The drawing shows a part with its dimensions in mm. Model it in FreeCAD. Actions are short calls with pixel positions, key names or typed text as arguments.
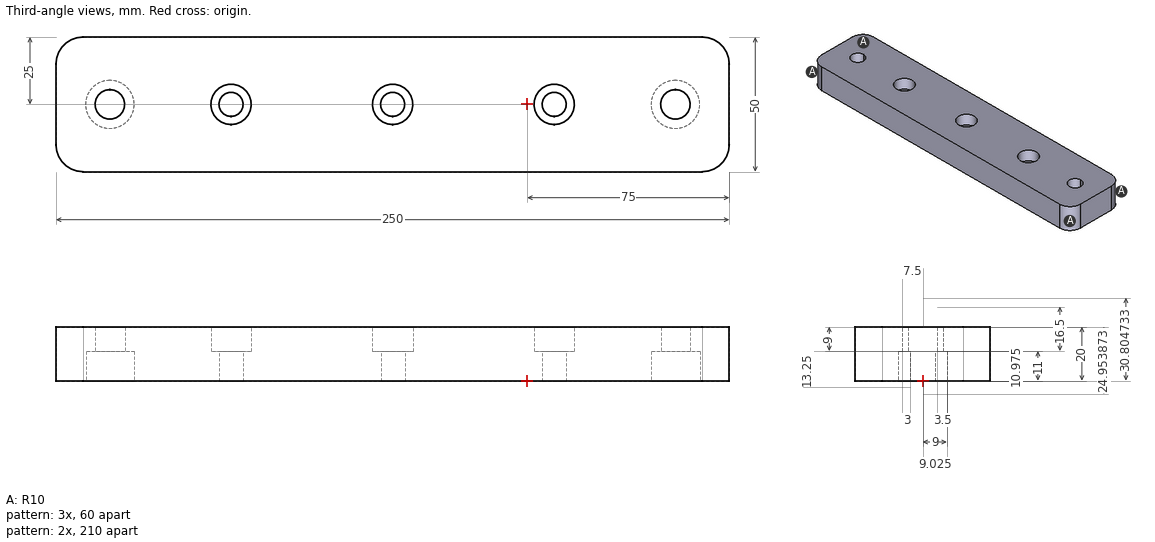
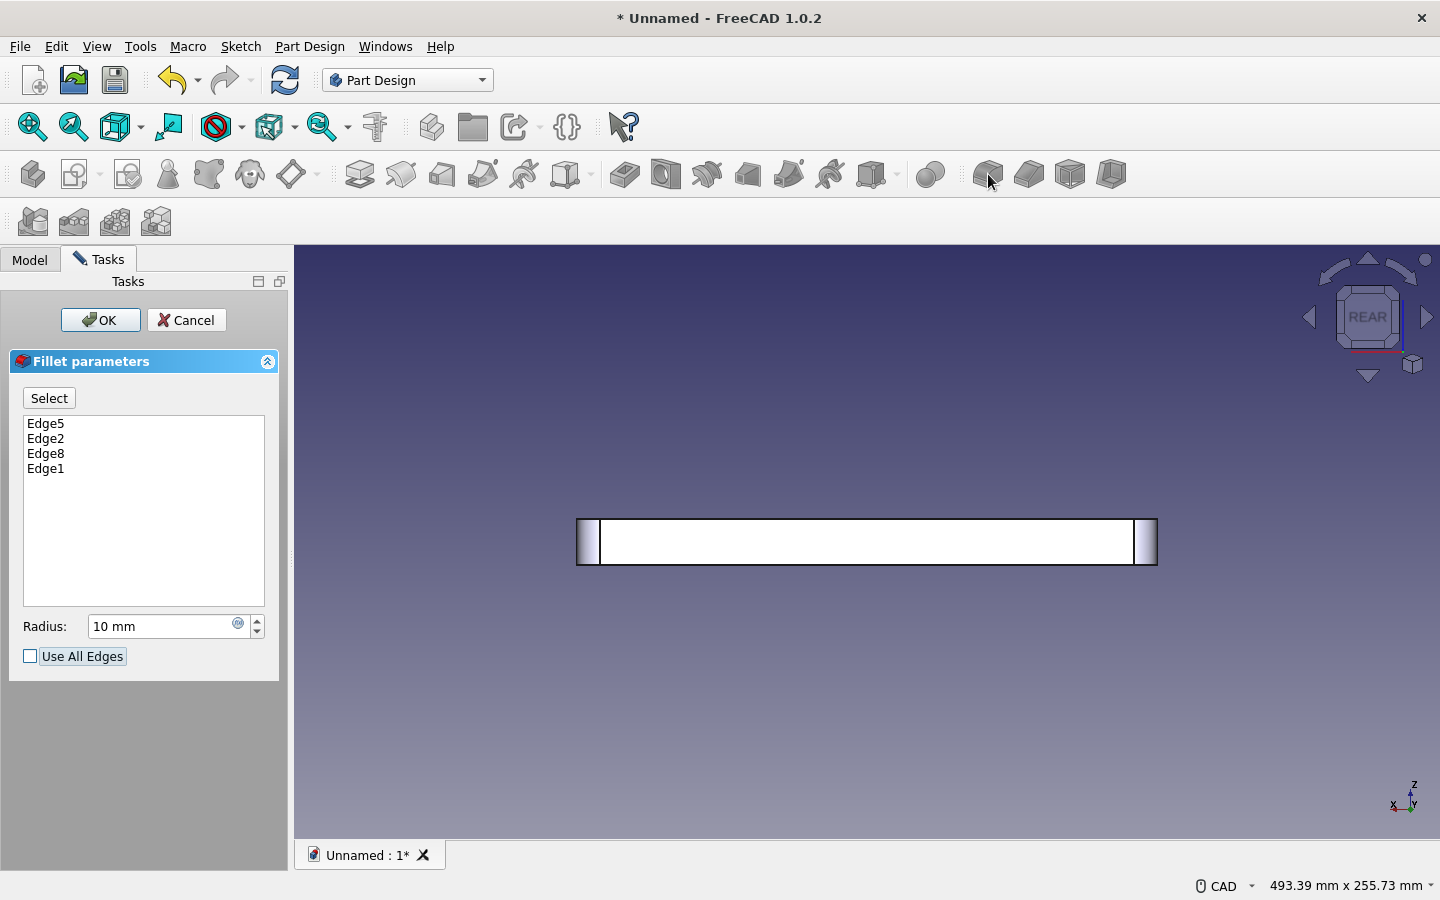
click(101, 320)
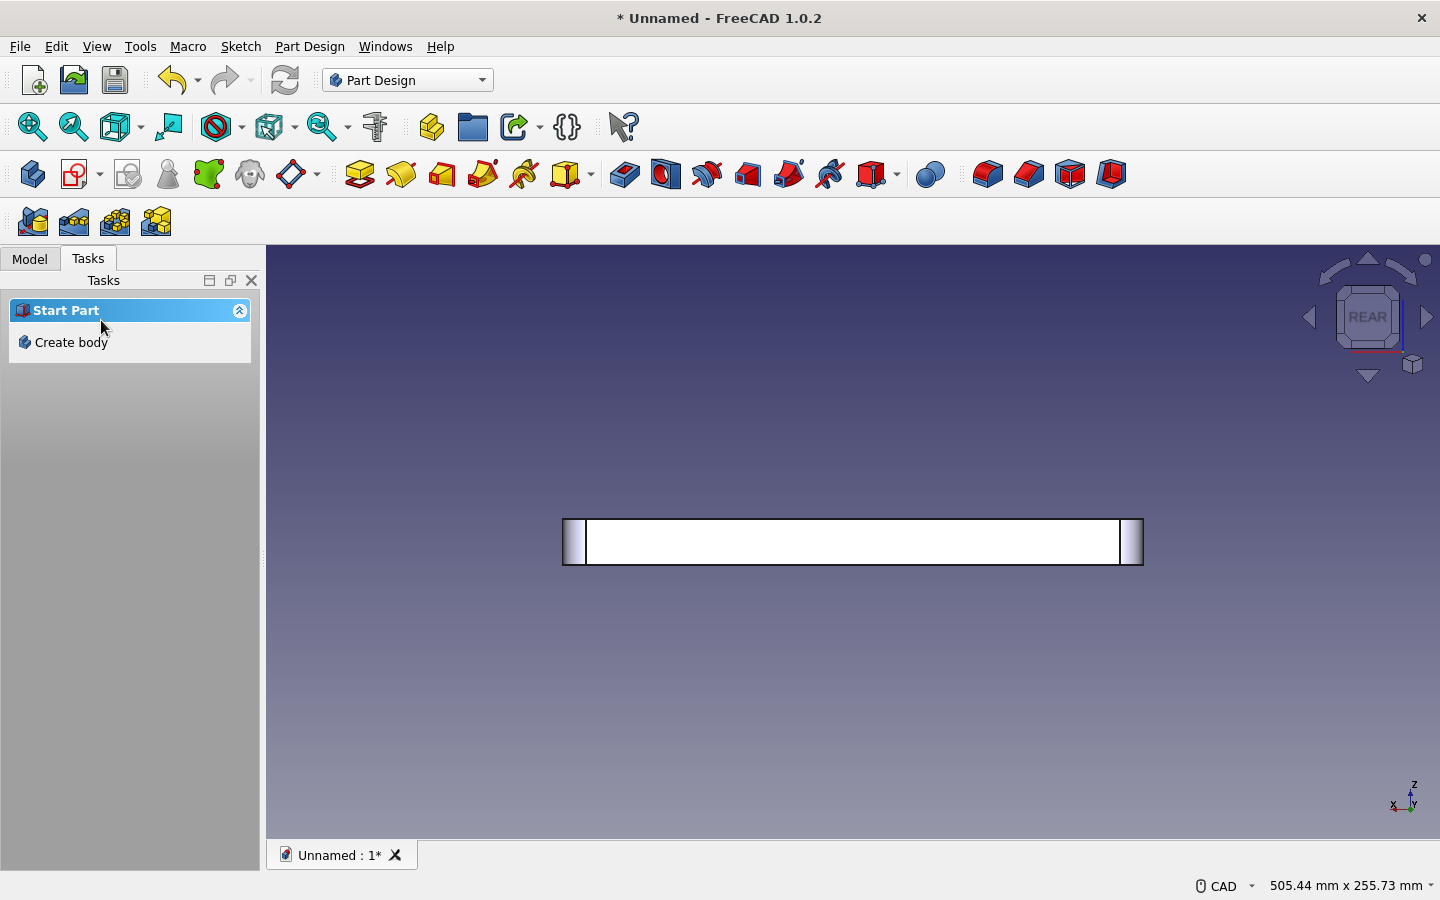
click(30, 258)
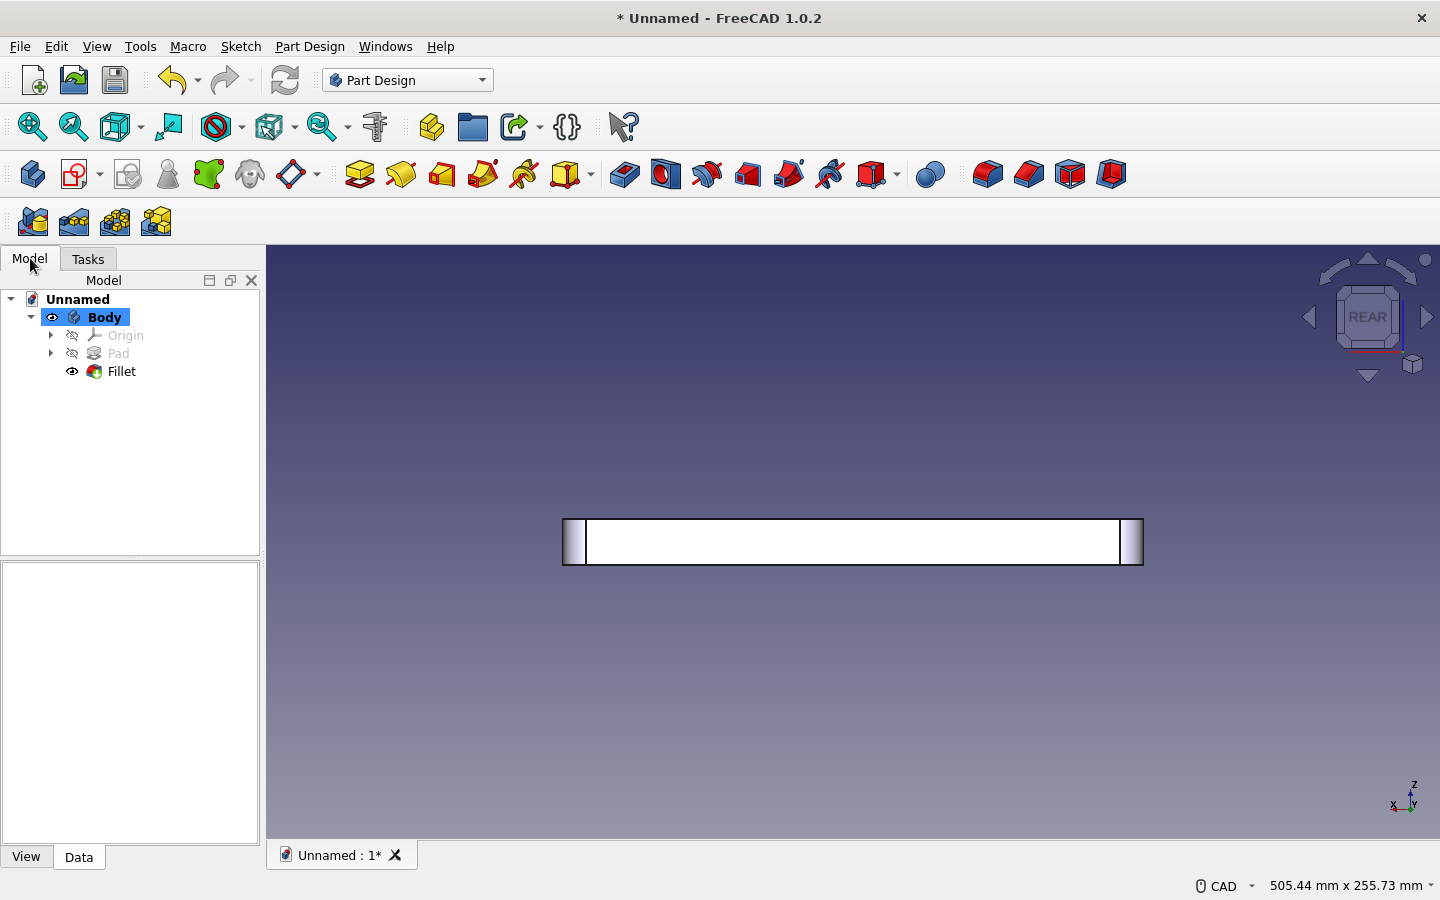
click(51, 335)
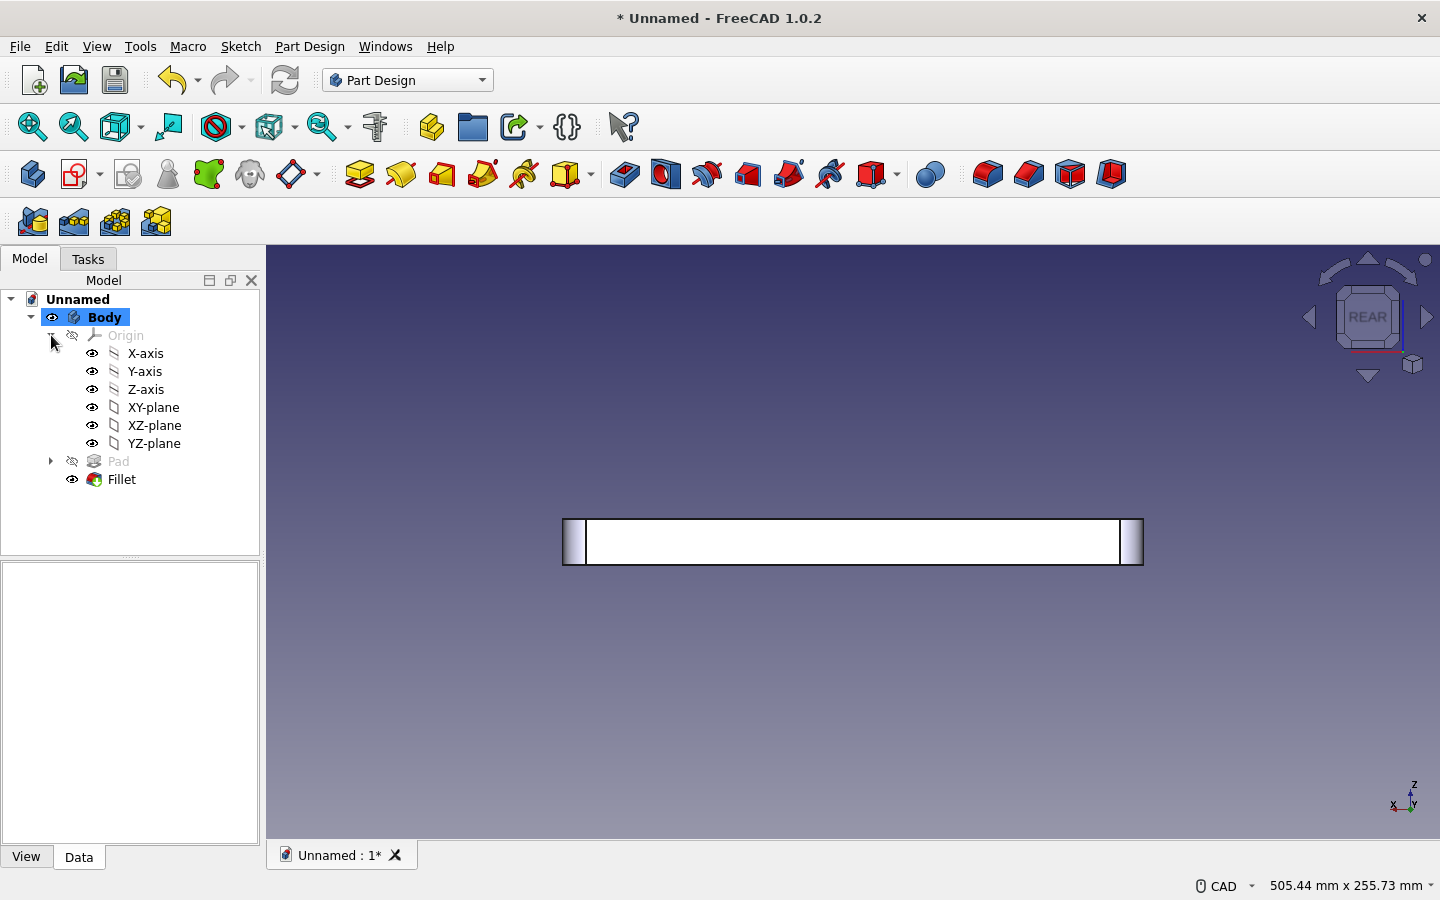
click(137, 443)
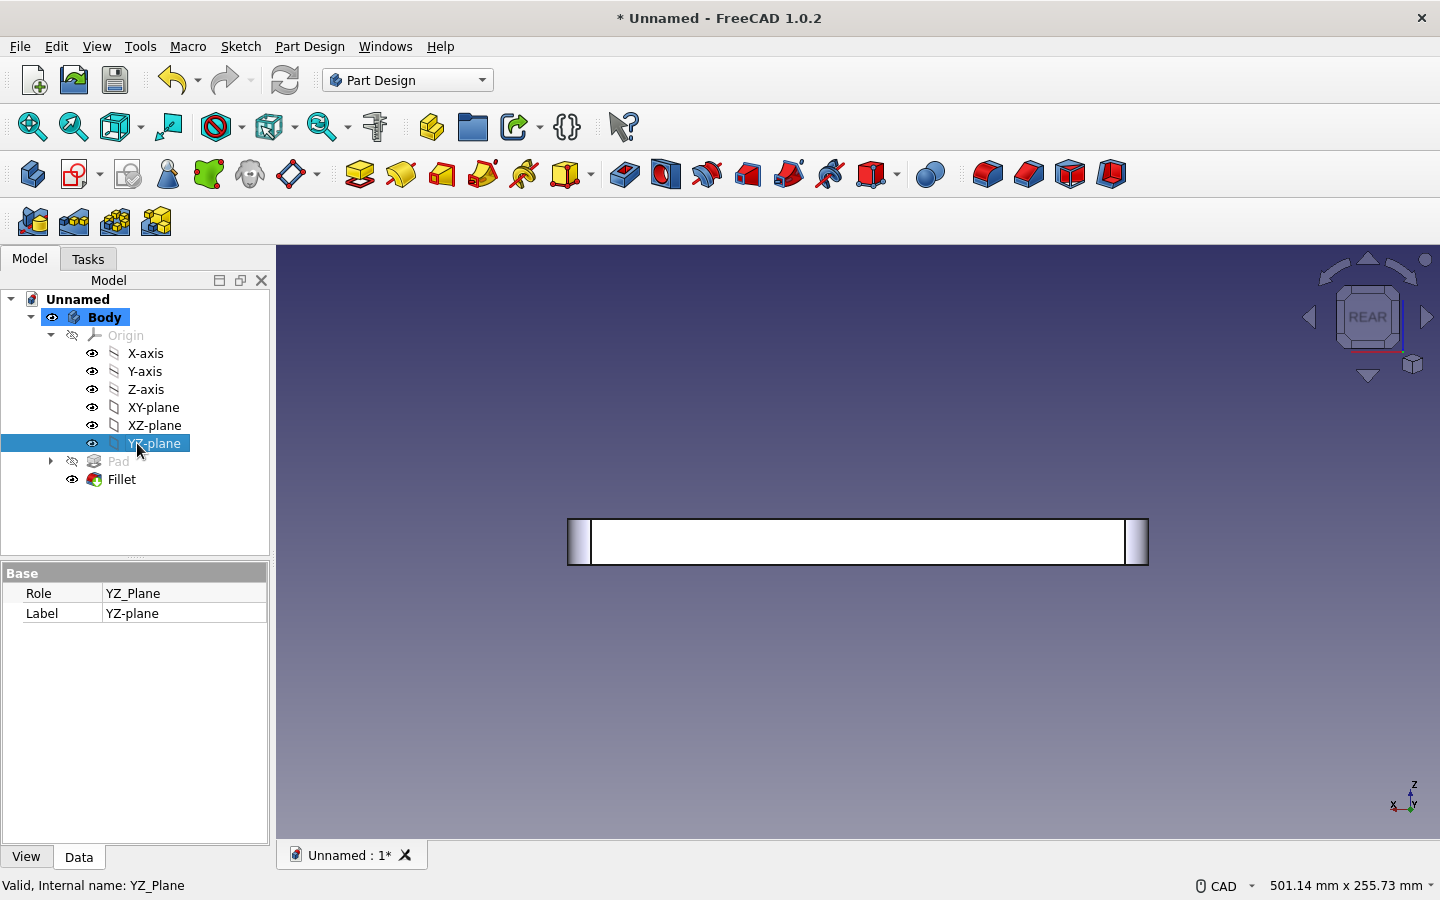
click(290, 174)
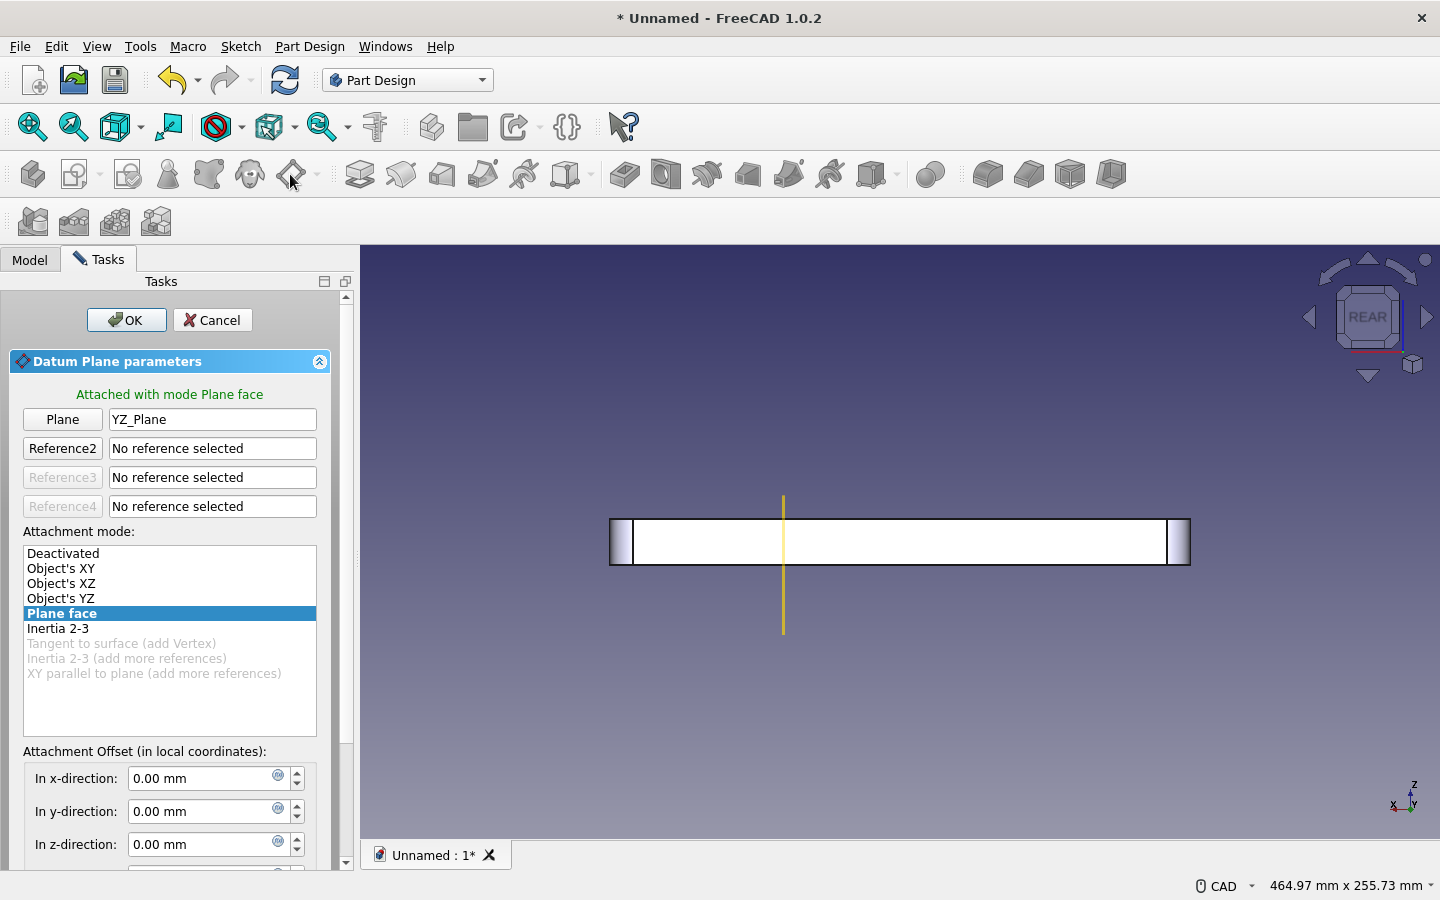
triple_click(210, 844)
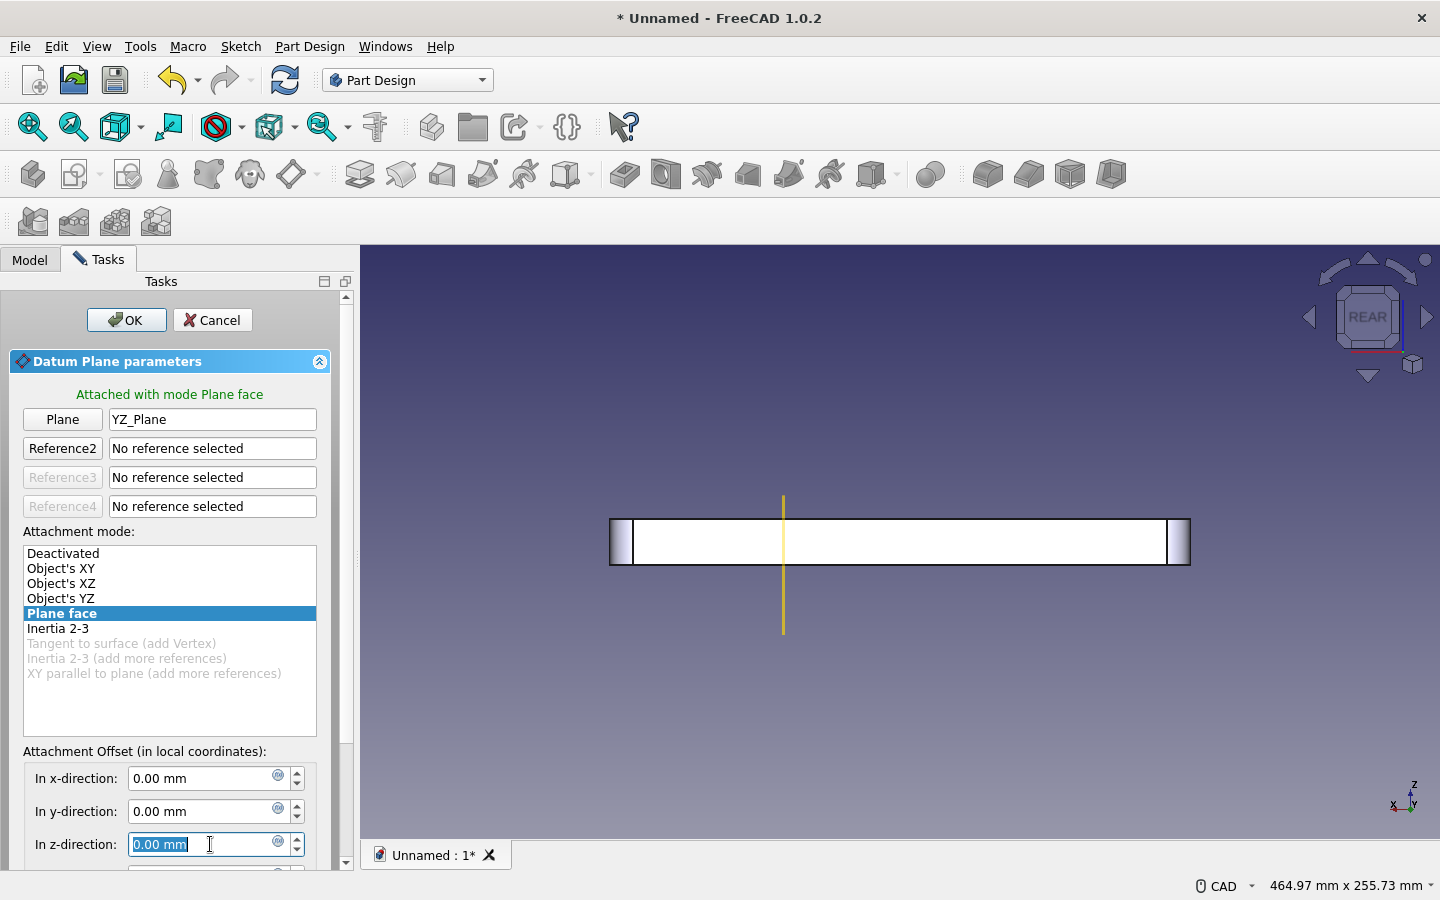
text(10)
key(Tab)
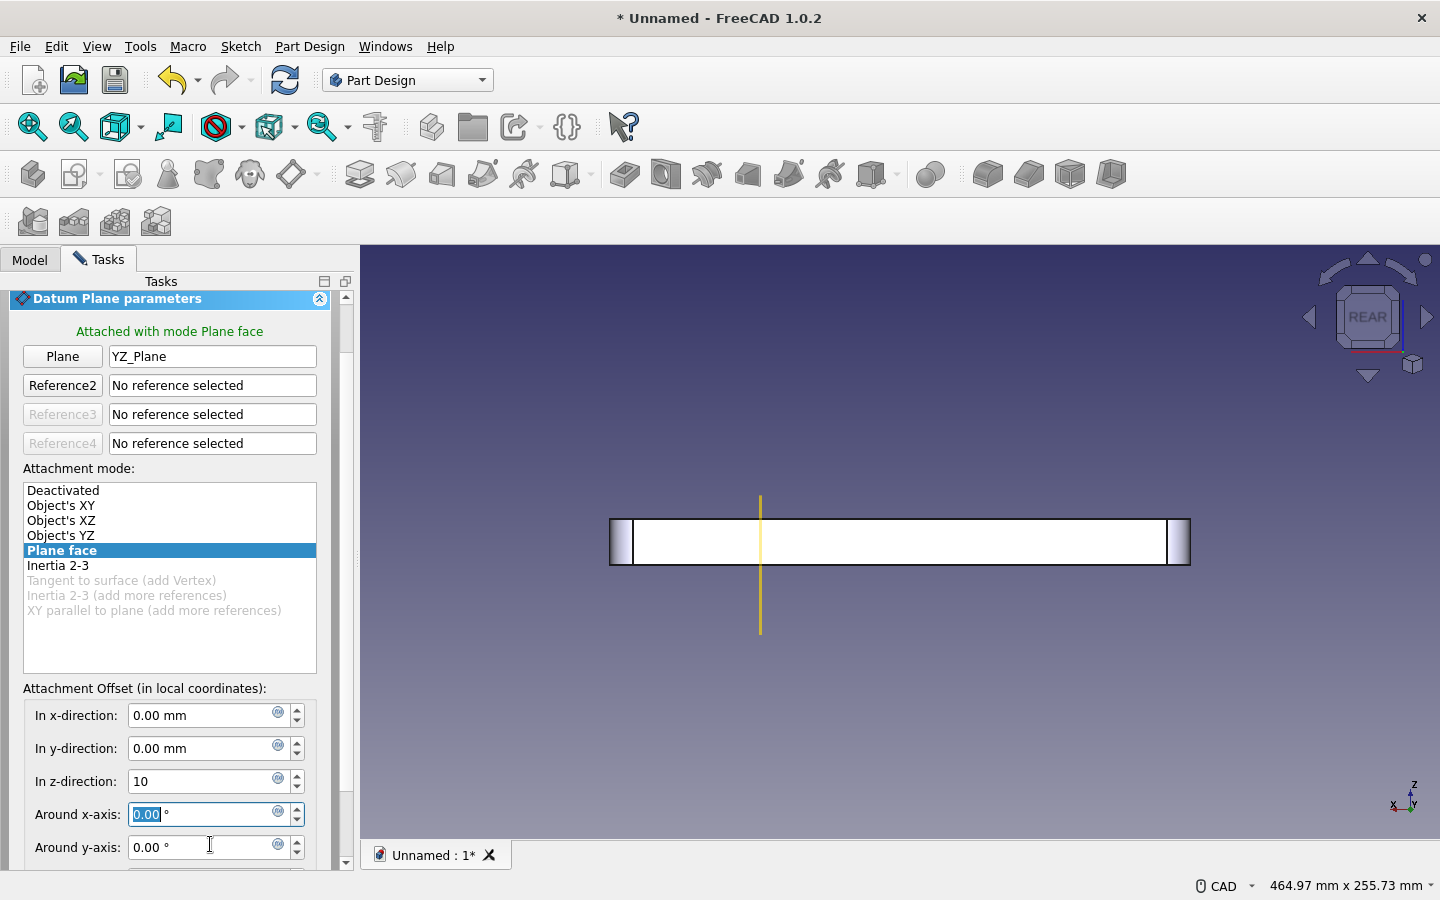
scroll(346, 580, up, 2)